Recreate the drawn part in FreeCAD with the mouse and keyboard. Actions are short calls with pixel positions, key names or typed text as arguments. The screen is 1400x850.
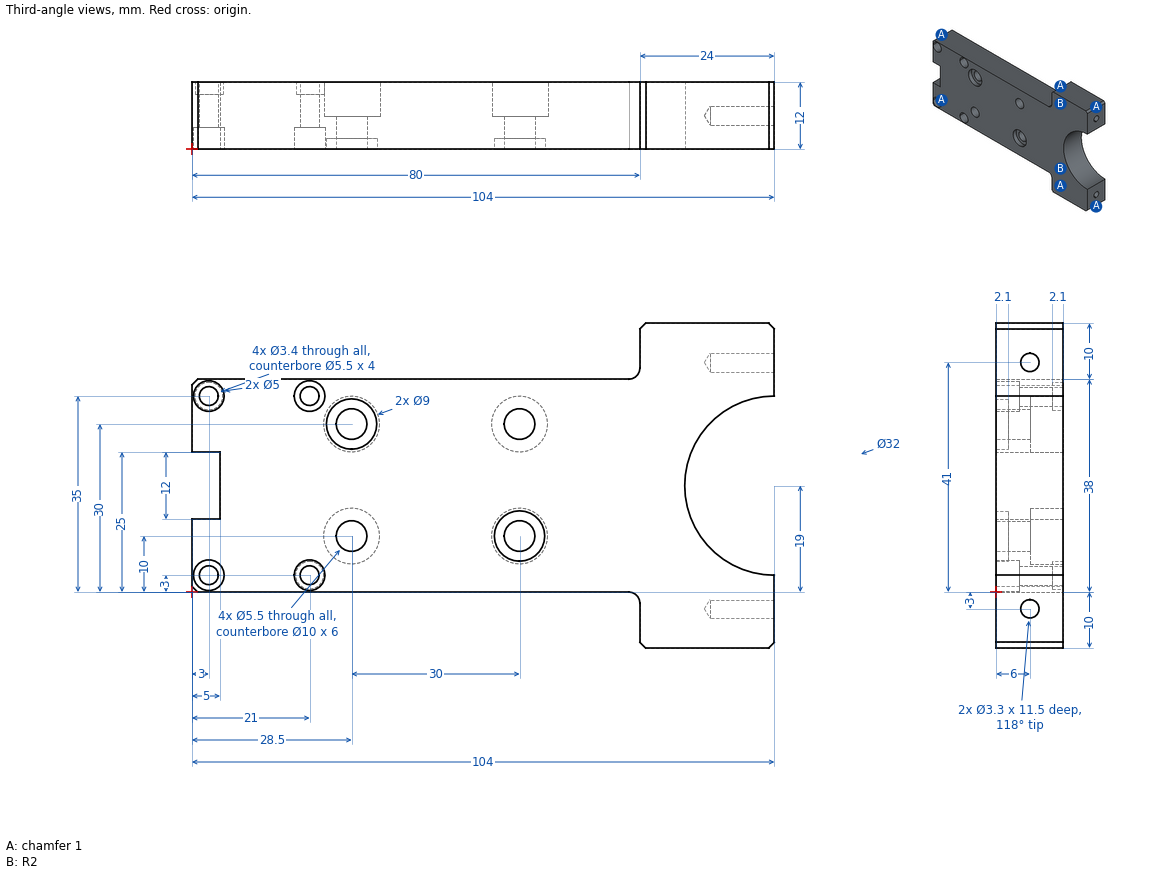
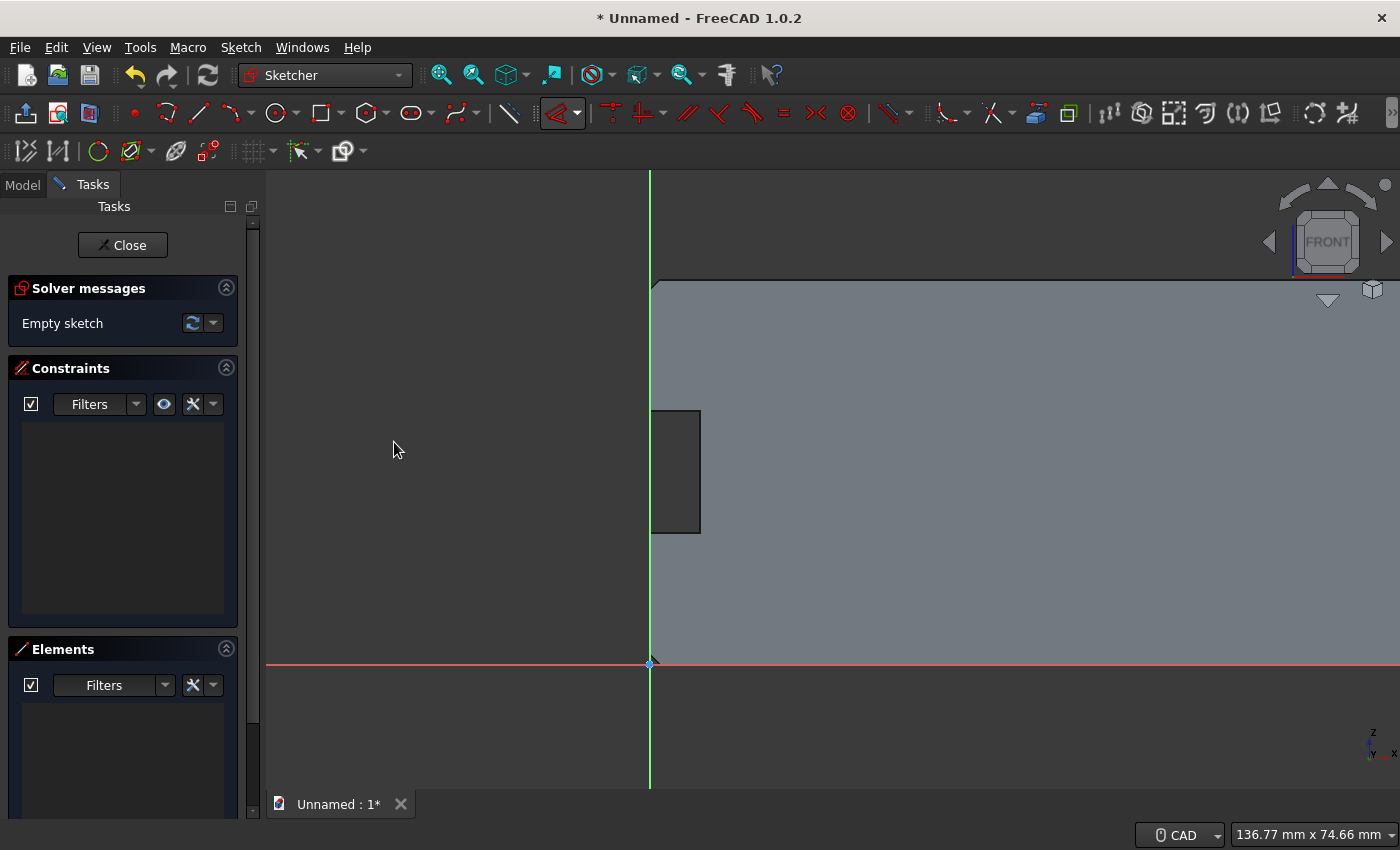
click(276, 114)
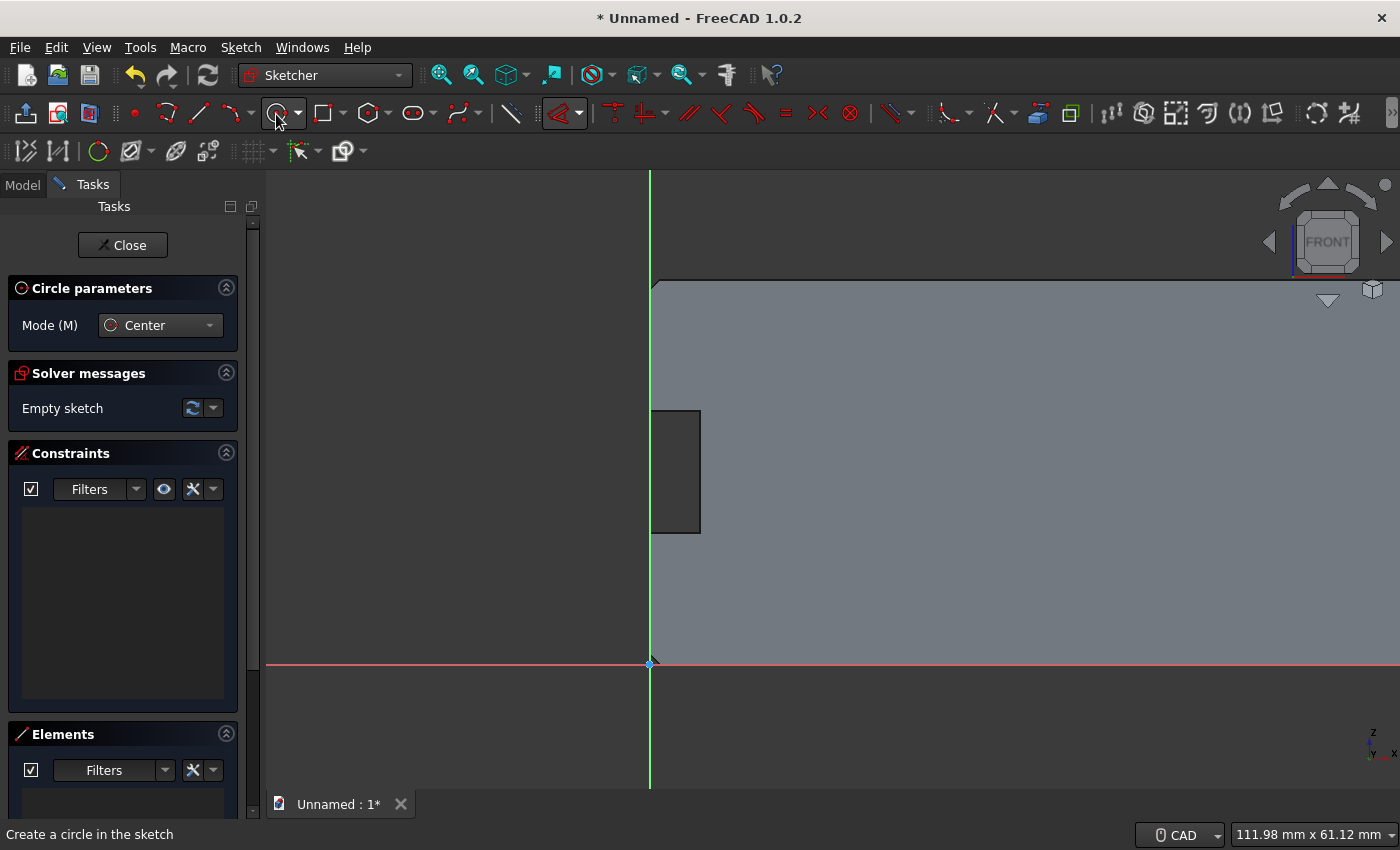
scroll(680, 310, up, 2)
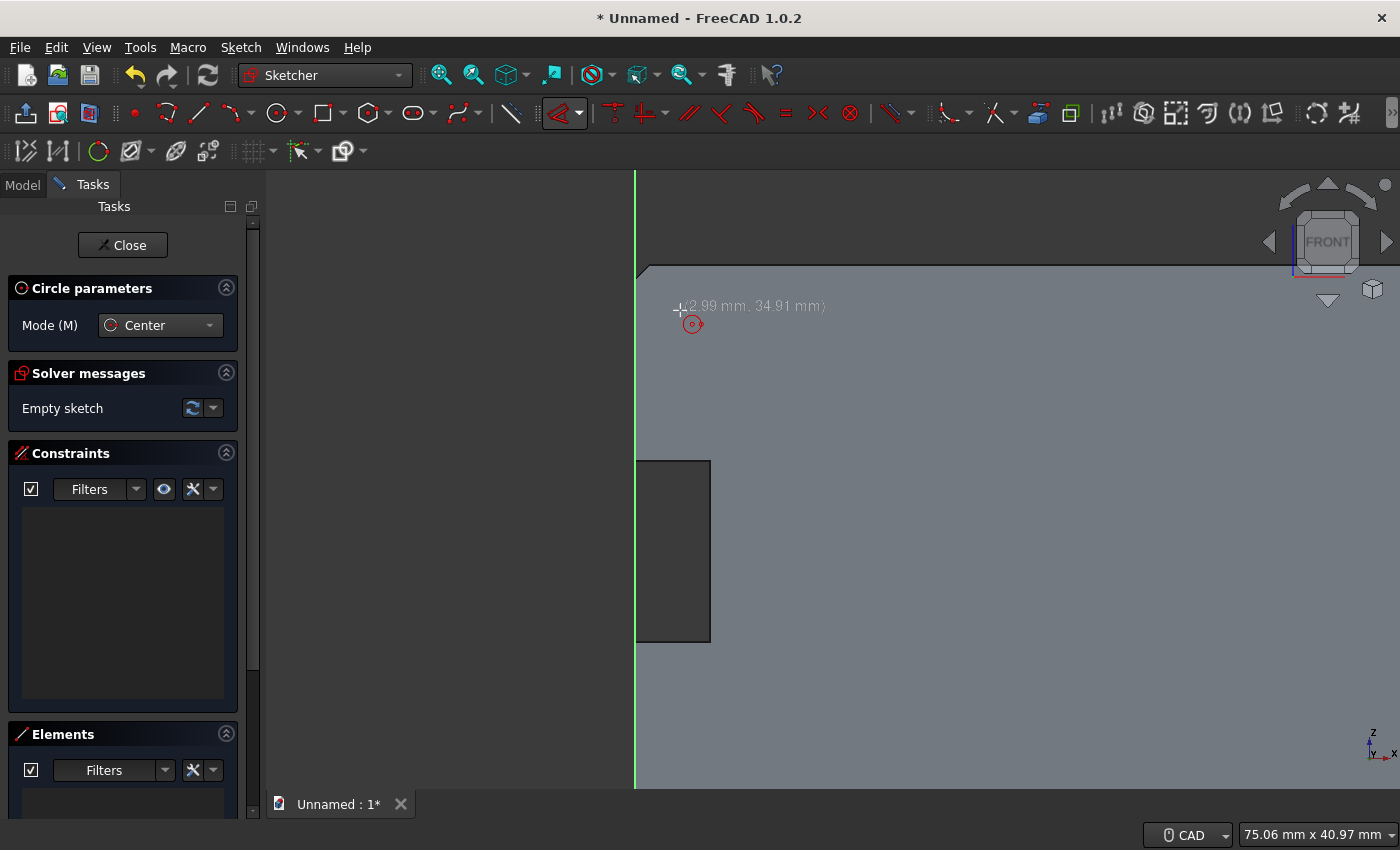
click(680, 310)
click(698, 292)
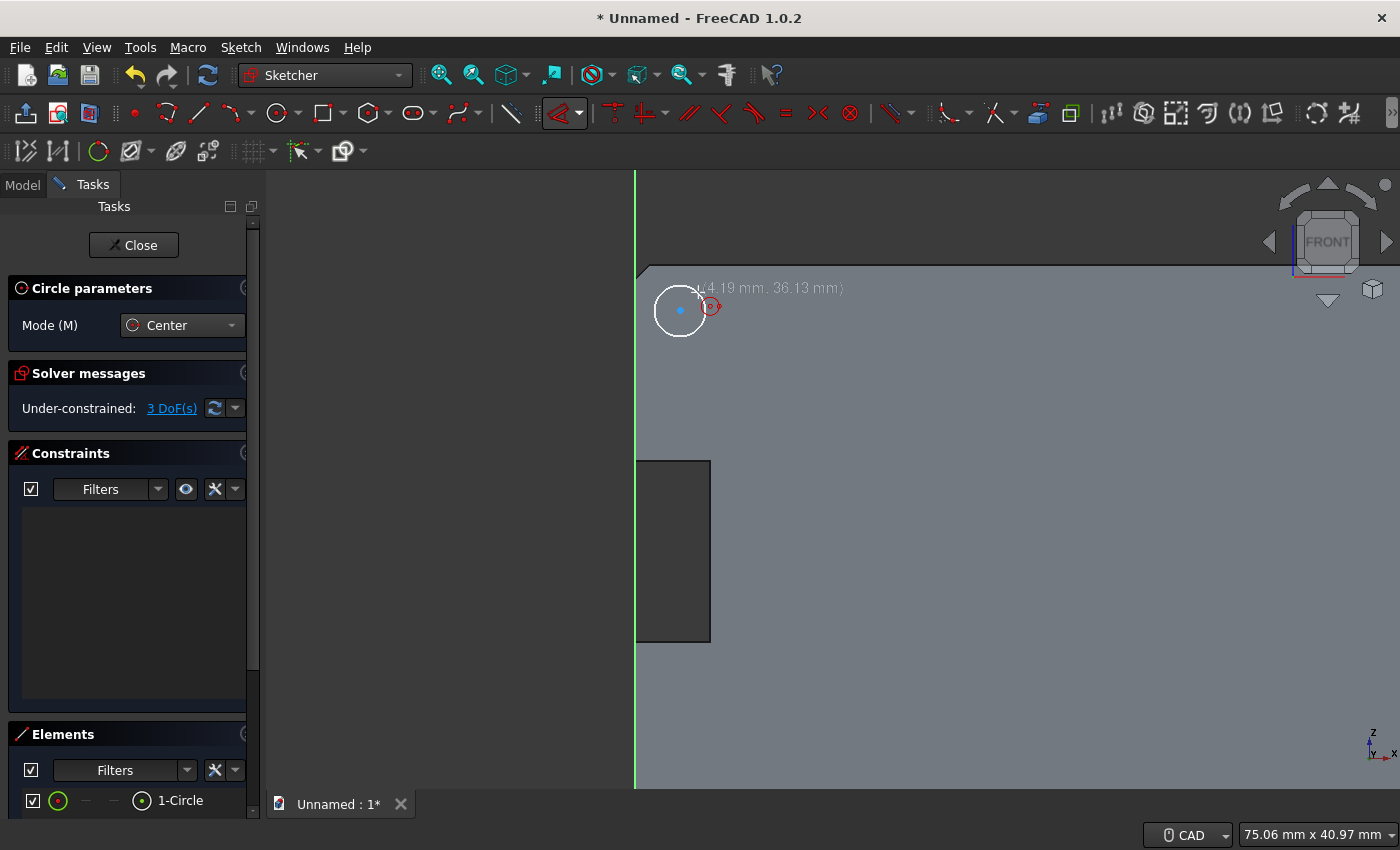
scroll(680, 312, down, 2)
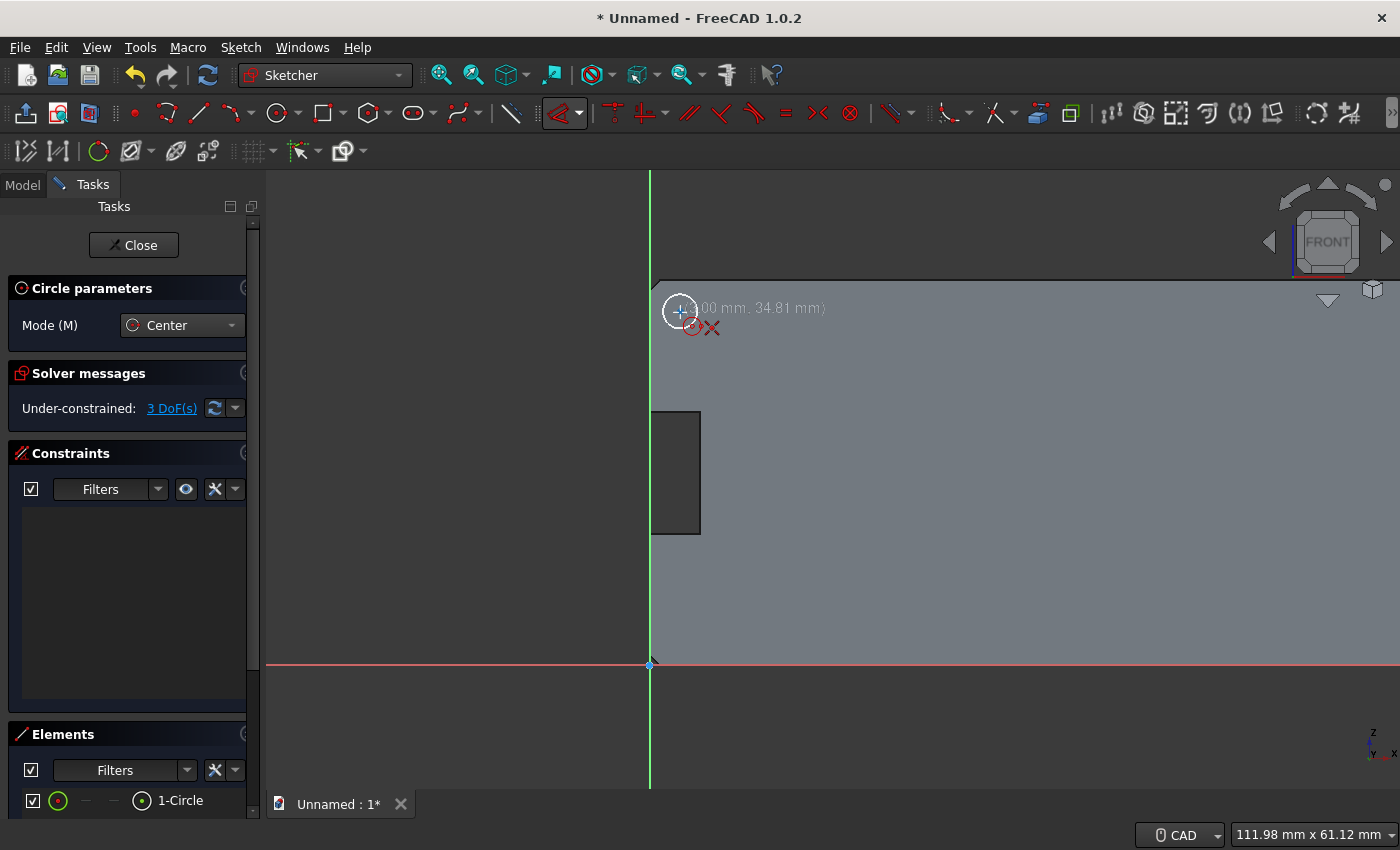
scroll(862, 635, up, 2)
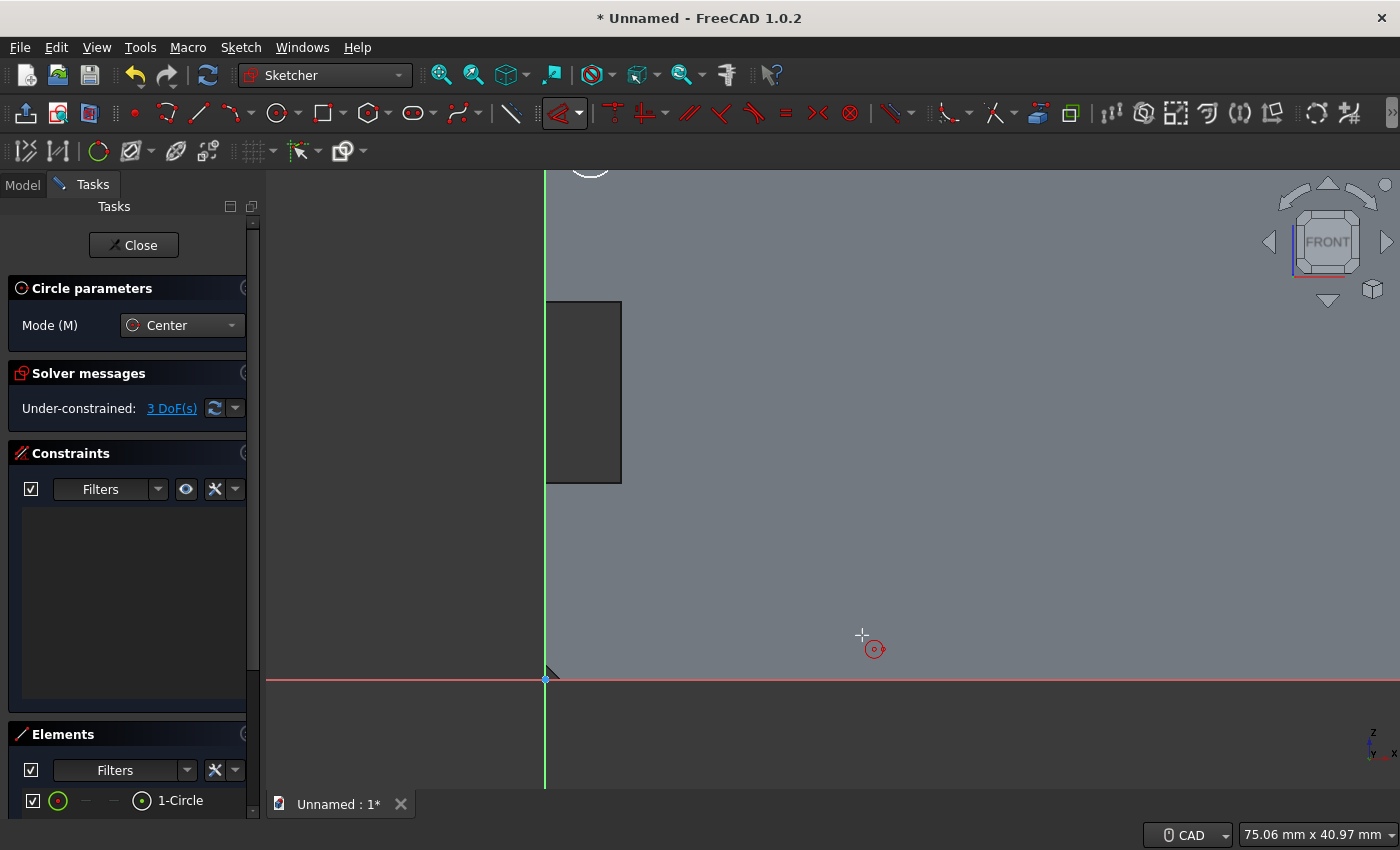
click(862, 634)
click(881, 616)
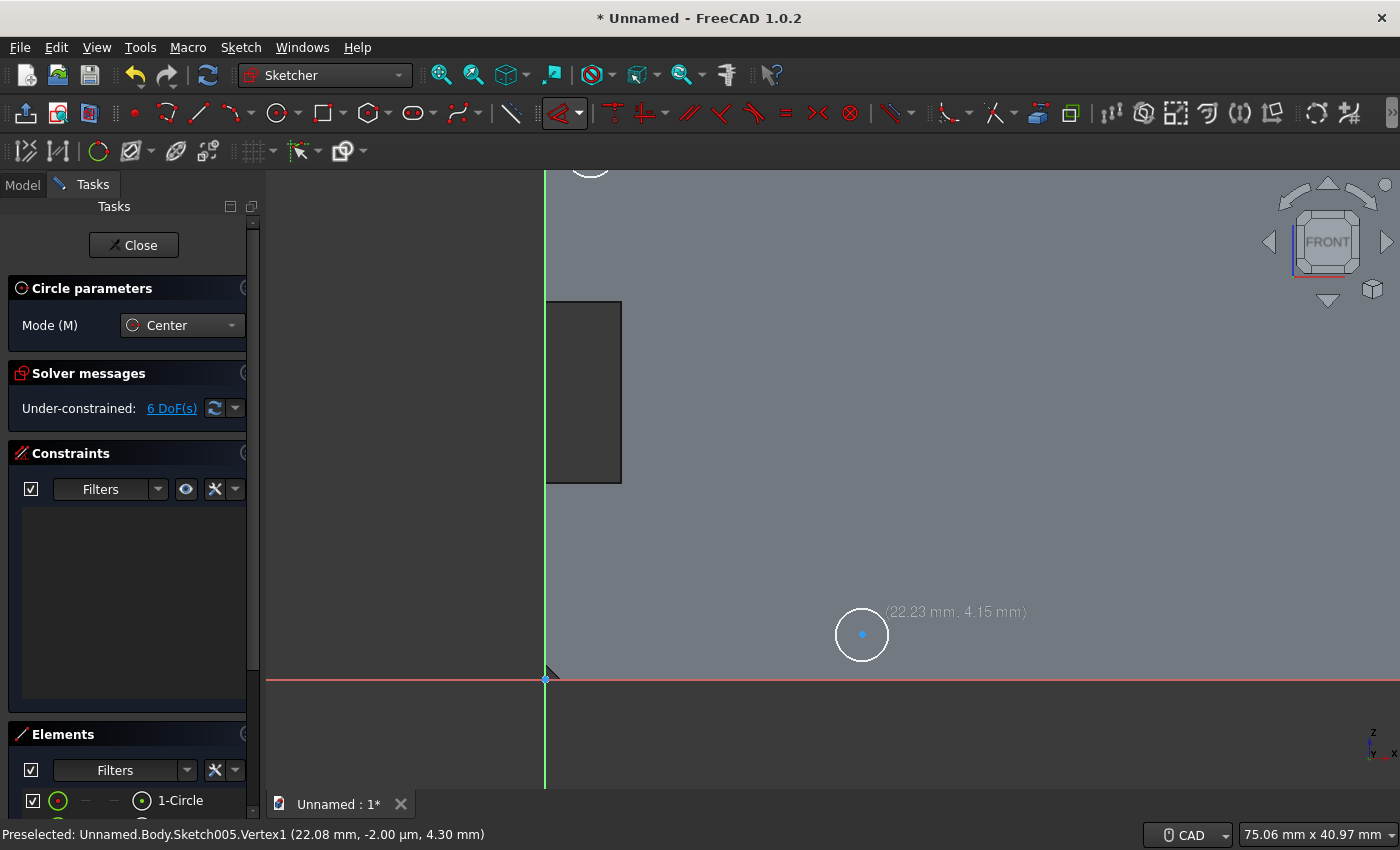
click(590, 634)
click(609, 616)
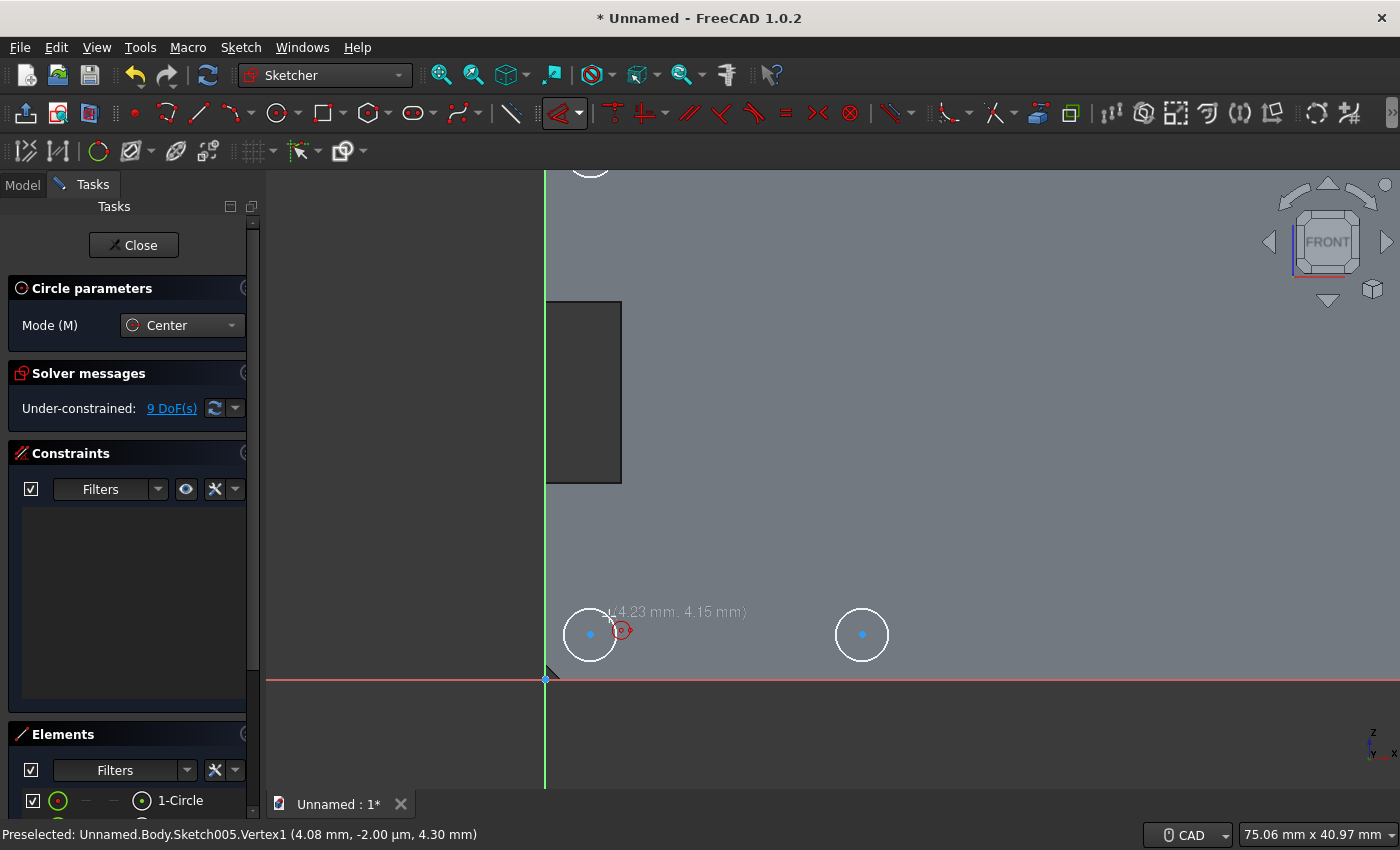
scroll(862, 636, down, 2)